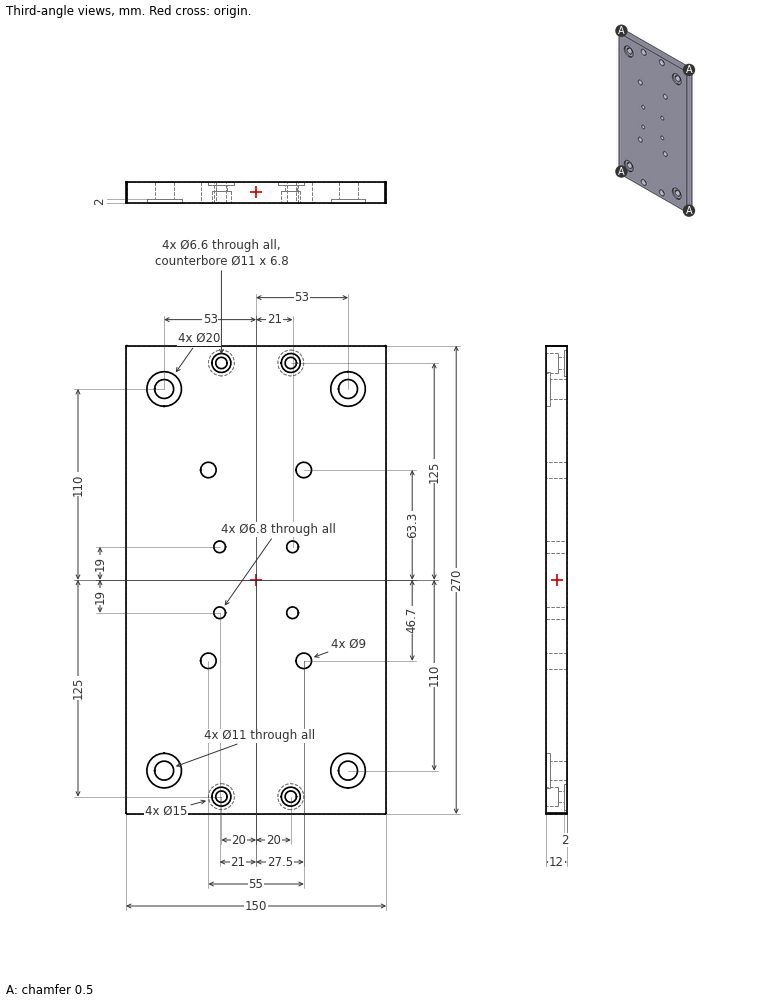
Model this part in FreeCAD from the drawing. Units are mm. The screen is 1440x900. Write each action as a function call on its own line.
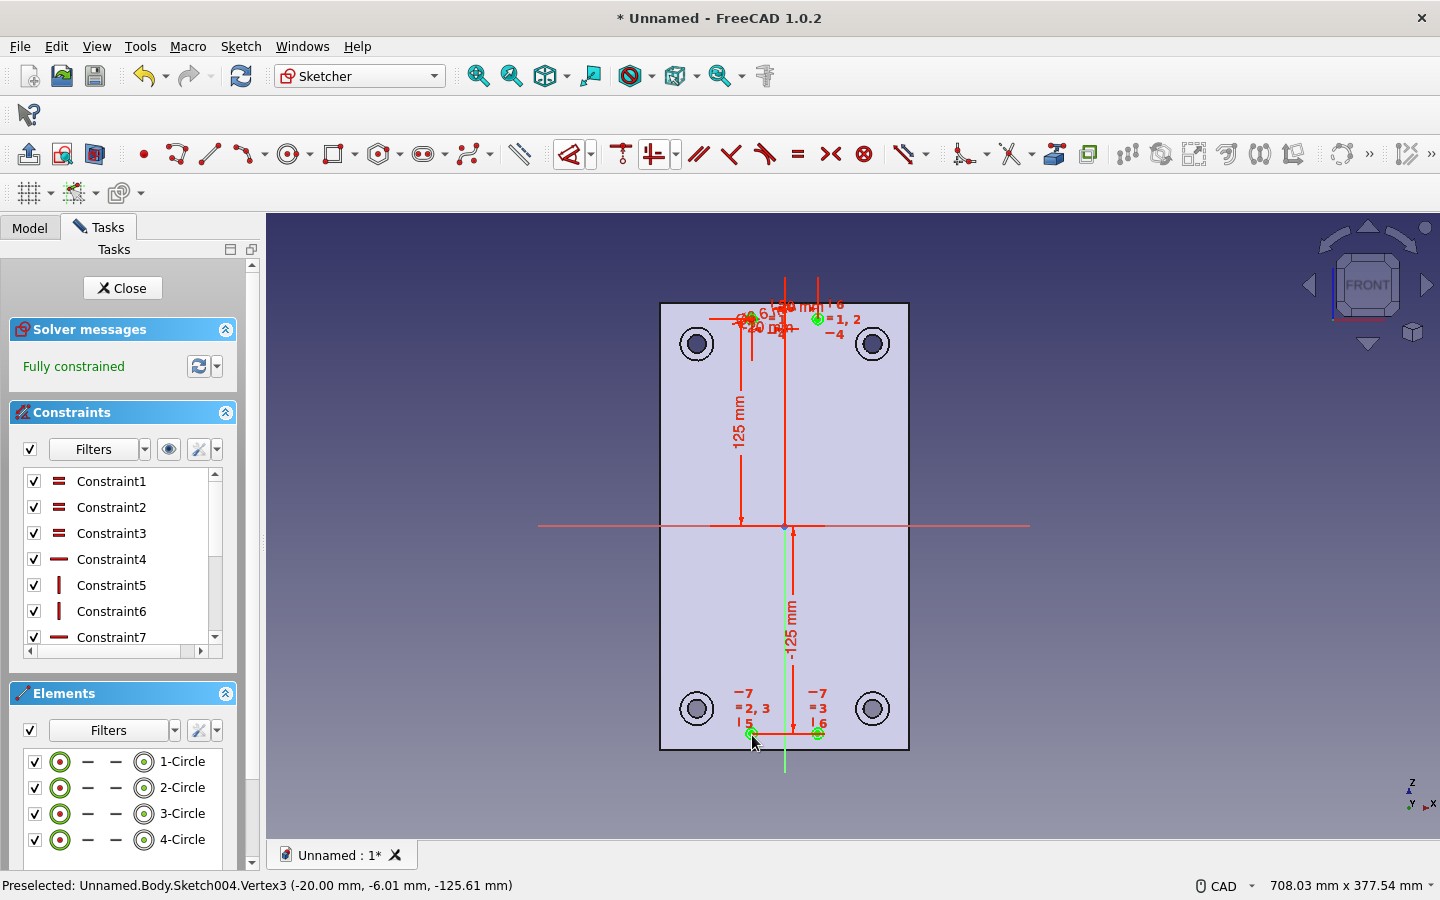
click(123, 288)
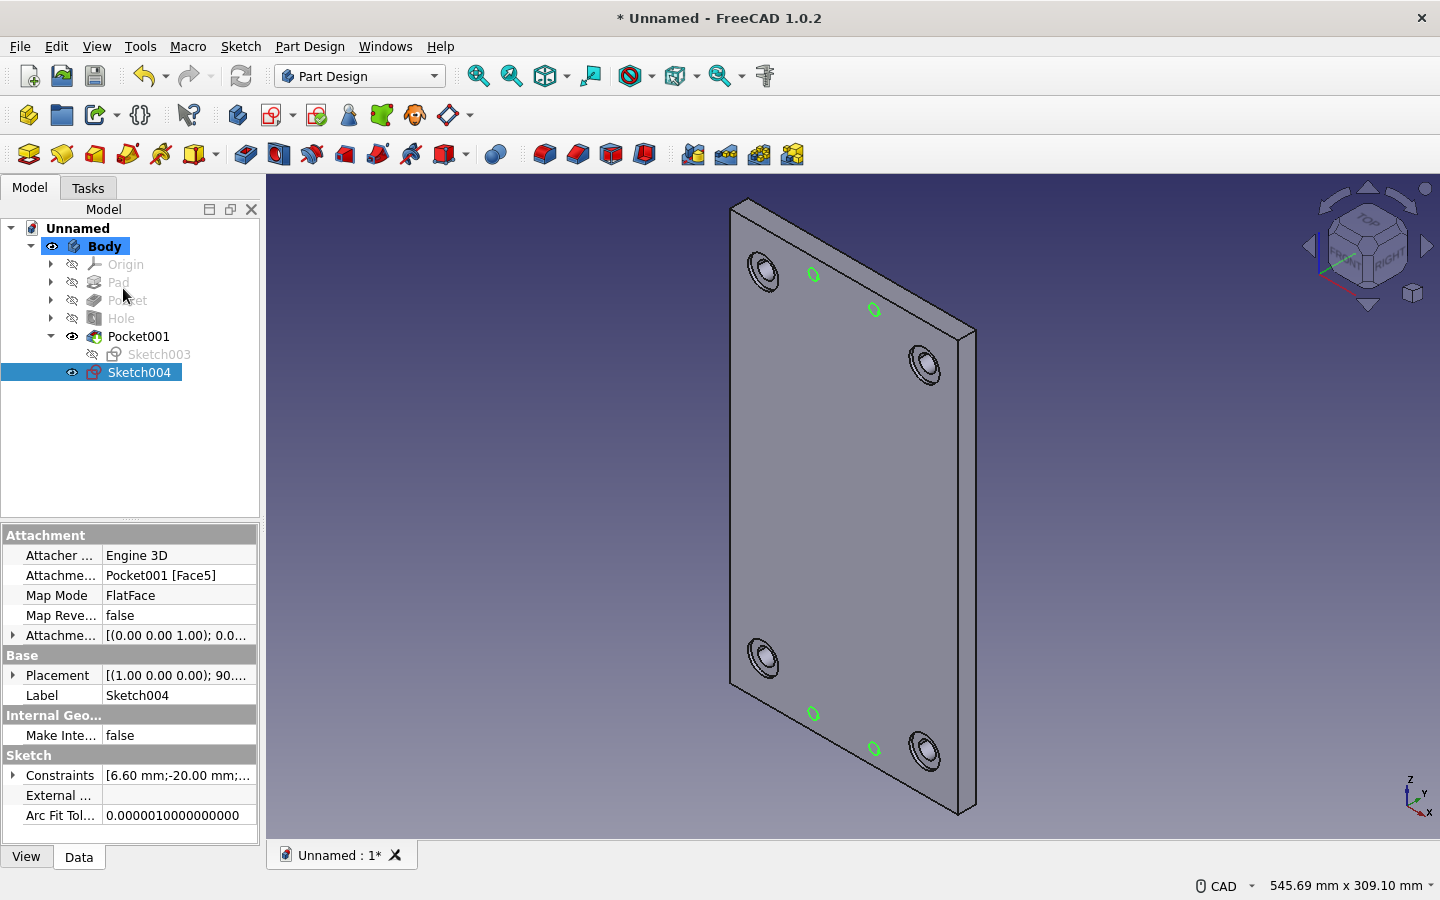
click(279, 154)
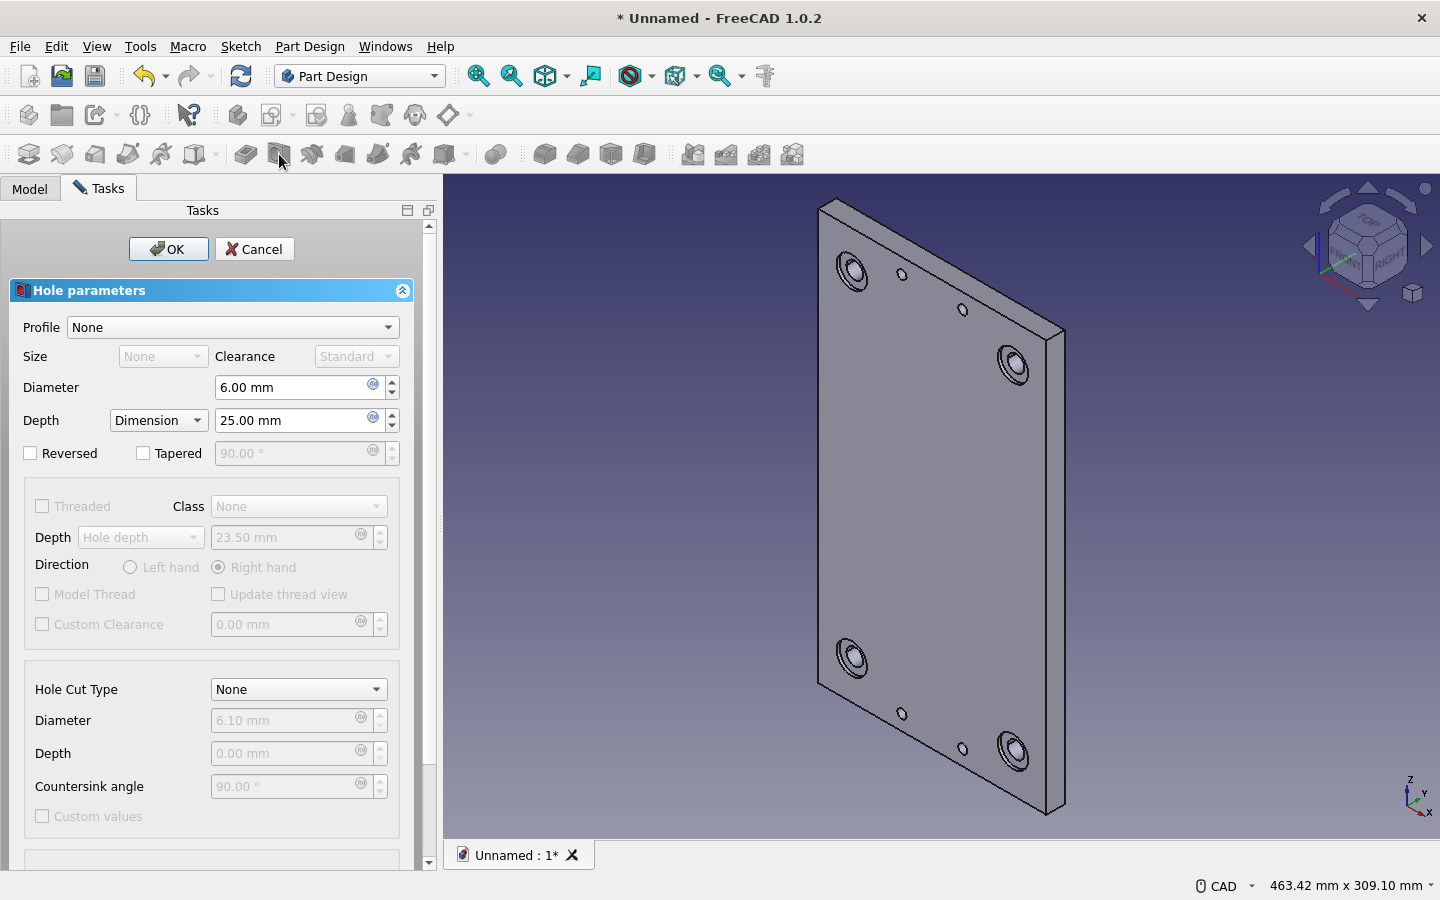
triple_click(300, 388)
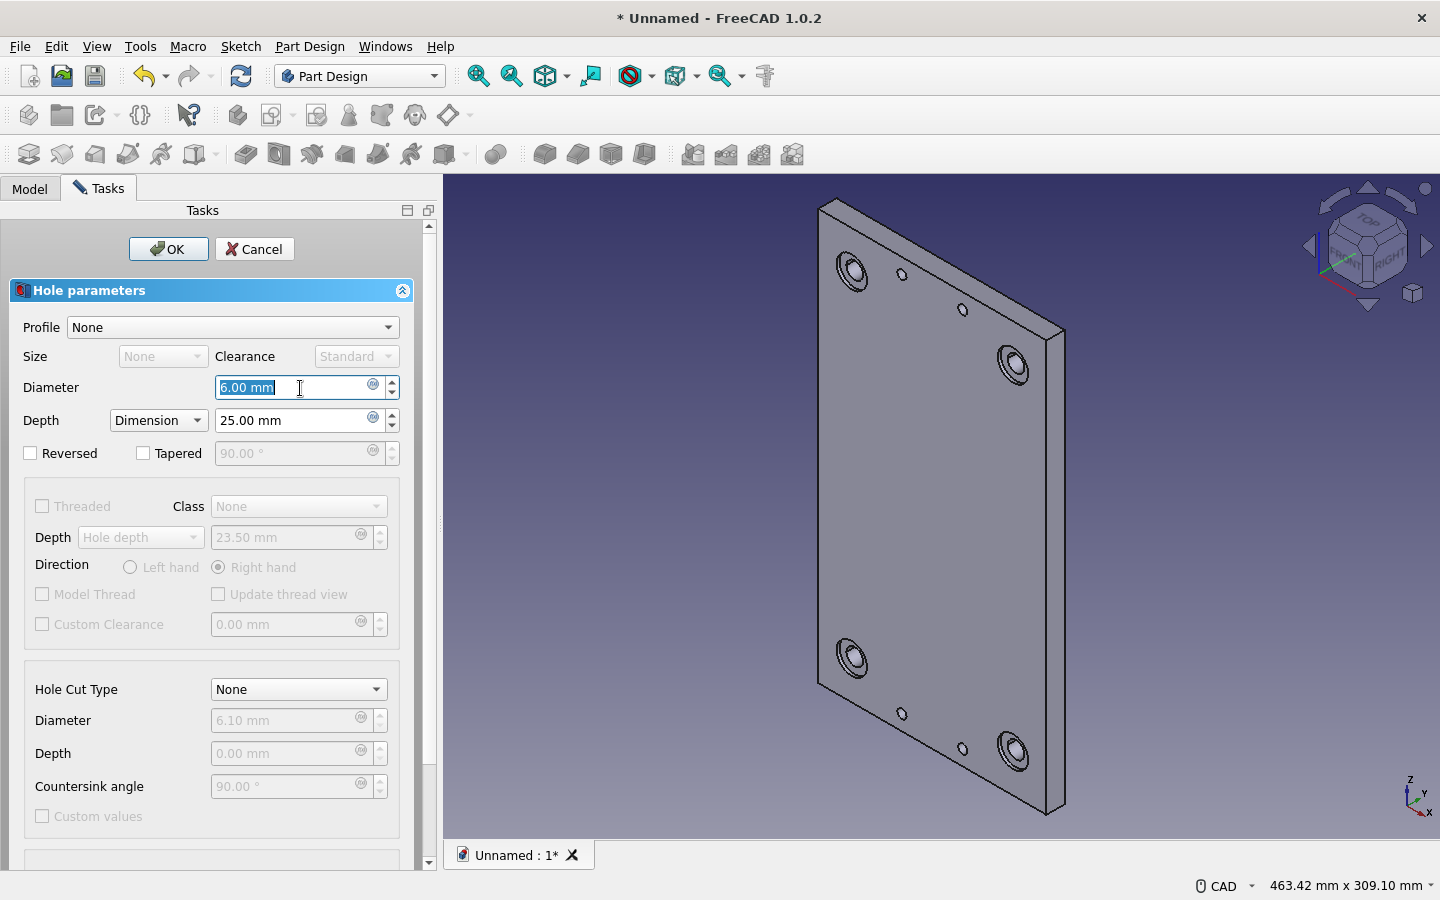
text(6.6)
key(Tab)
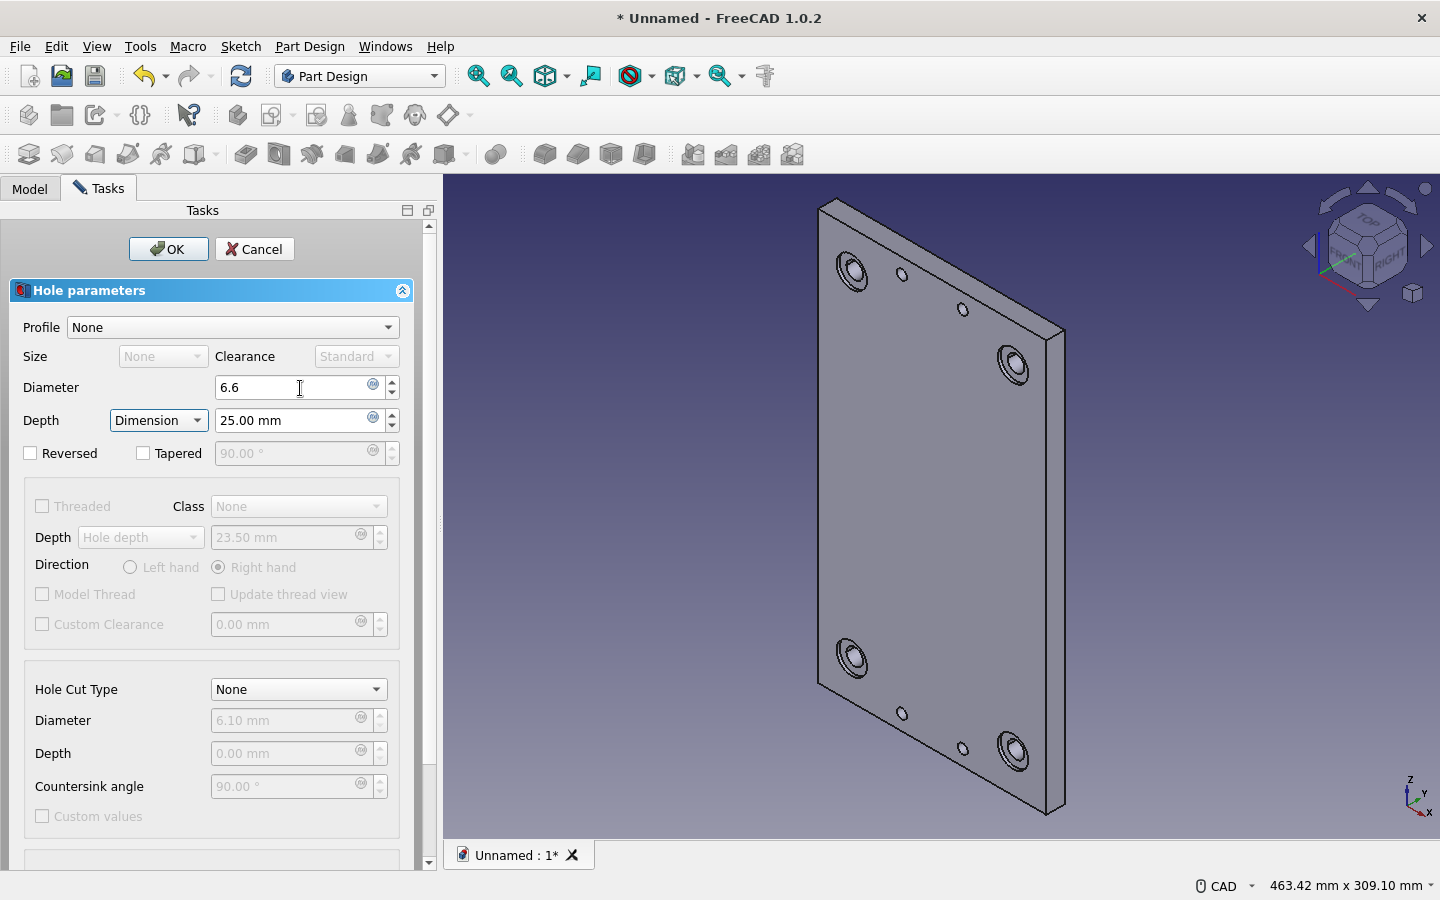
click(160, 420)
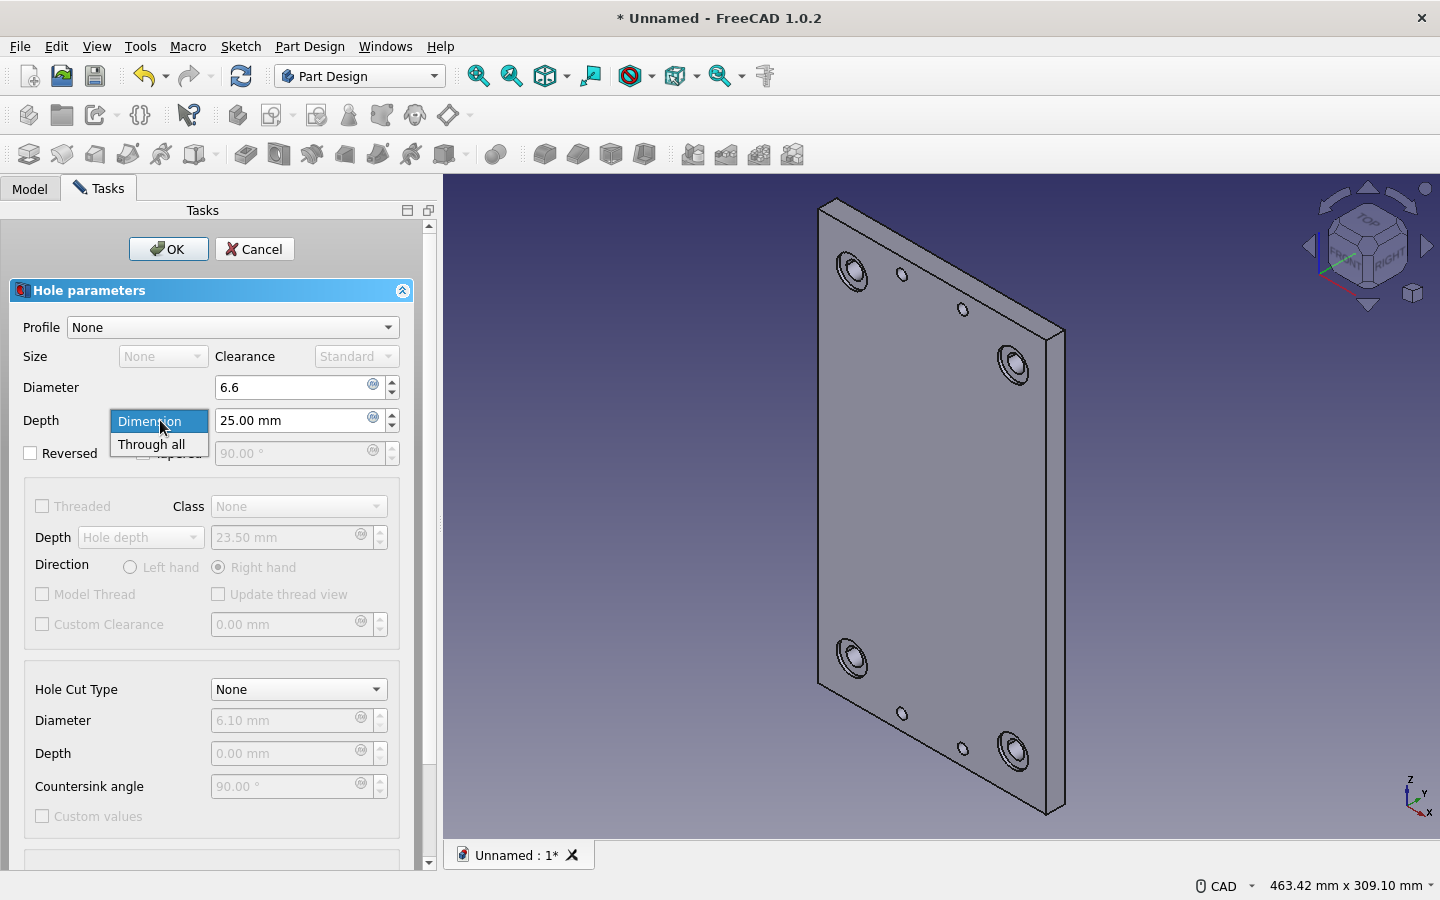
click(158, 444)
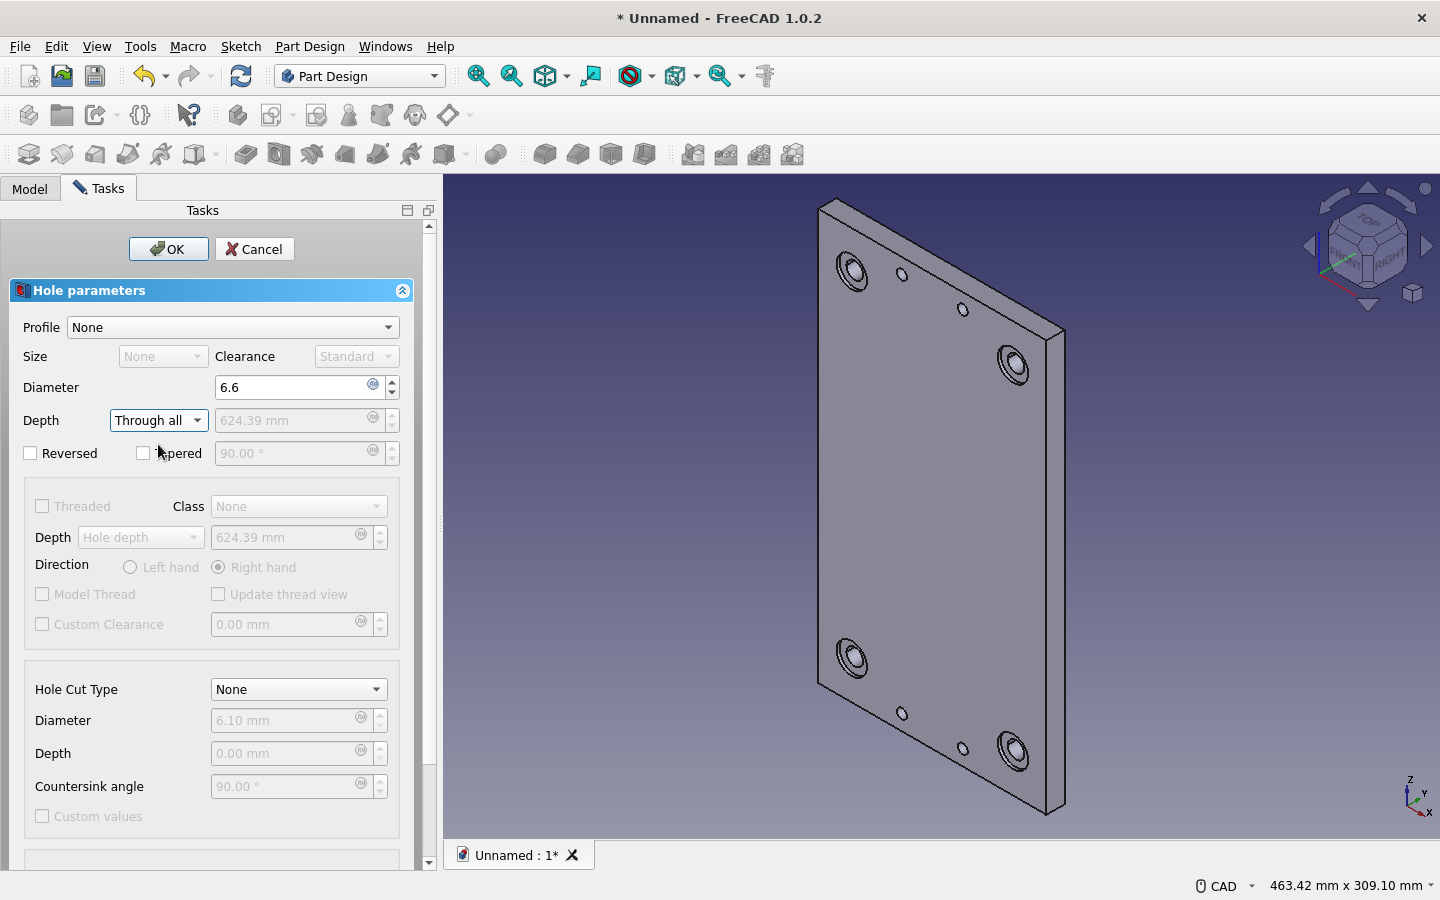
click(300, 690)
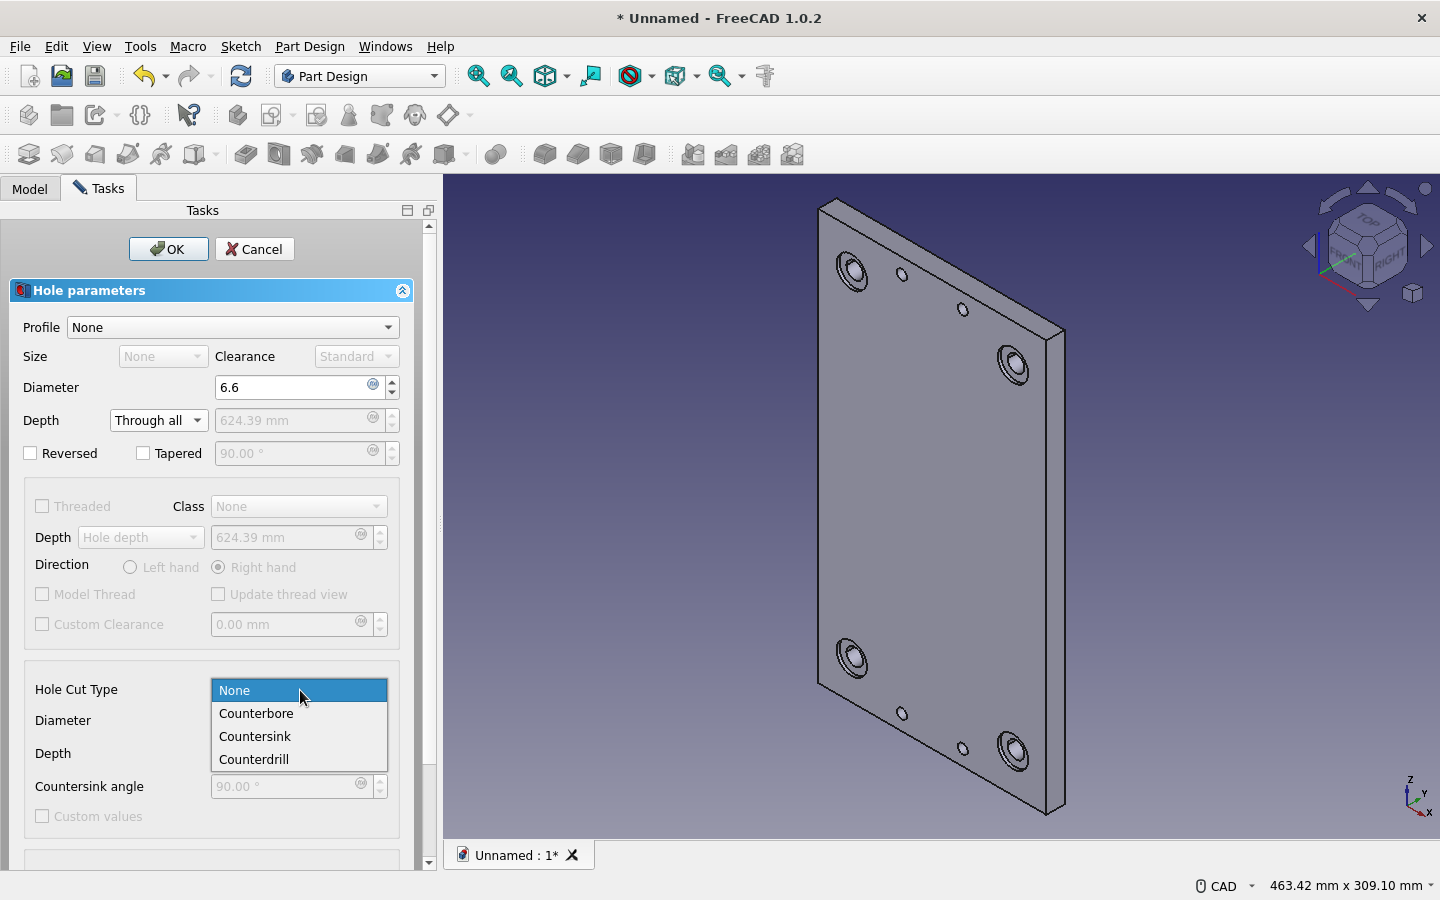
click(298, 714)